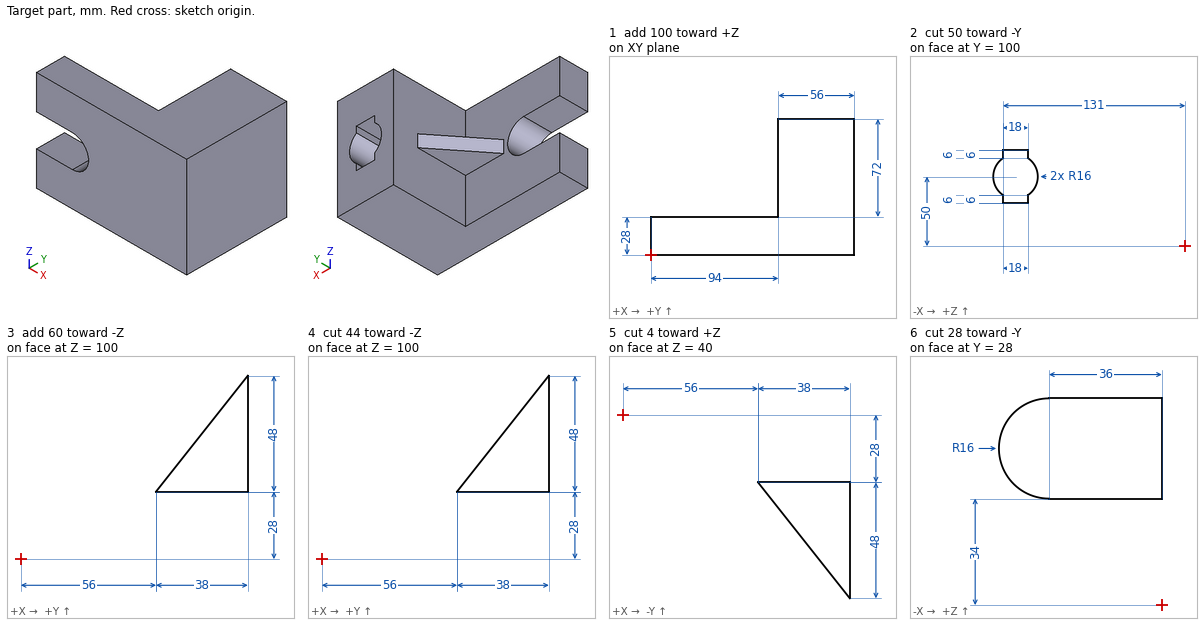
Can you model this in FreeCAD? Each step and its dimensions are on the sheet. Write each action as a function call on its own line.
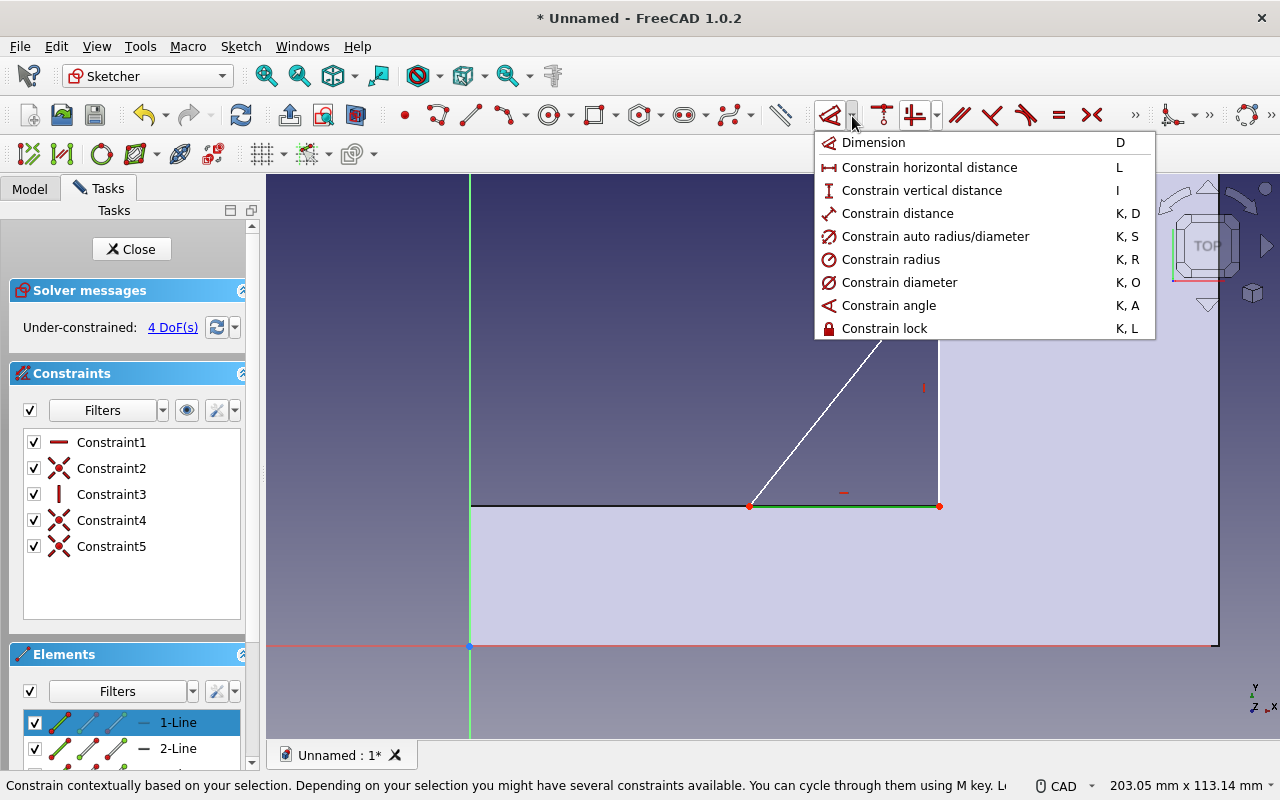
click(985, 168)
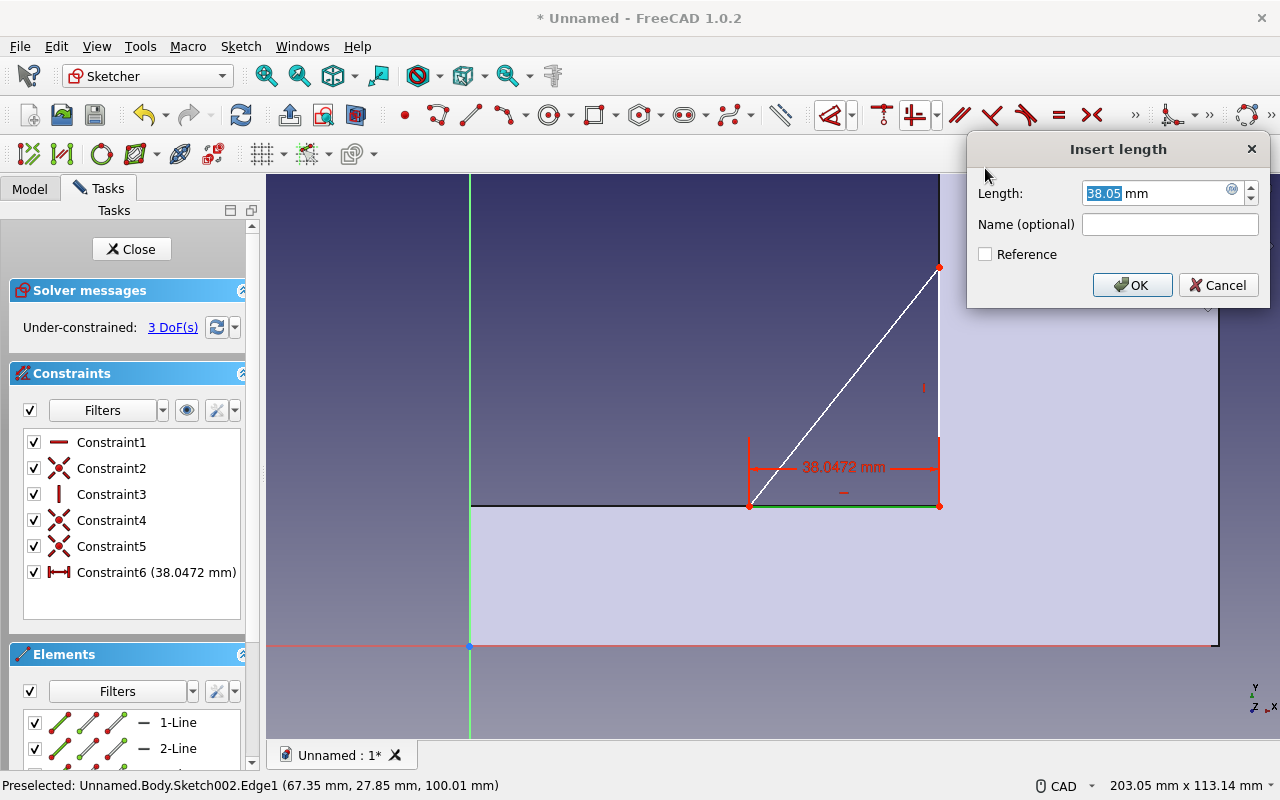
text(38)
key(Return)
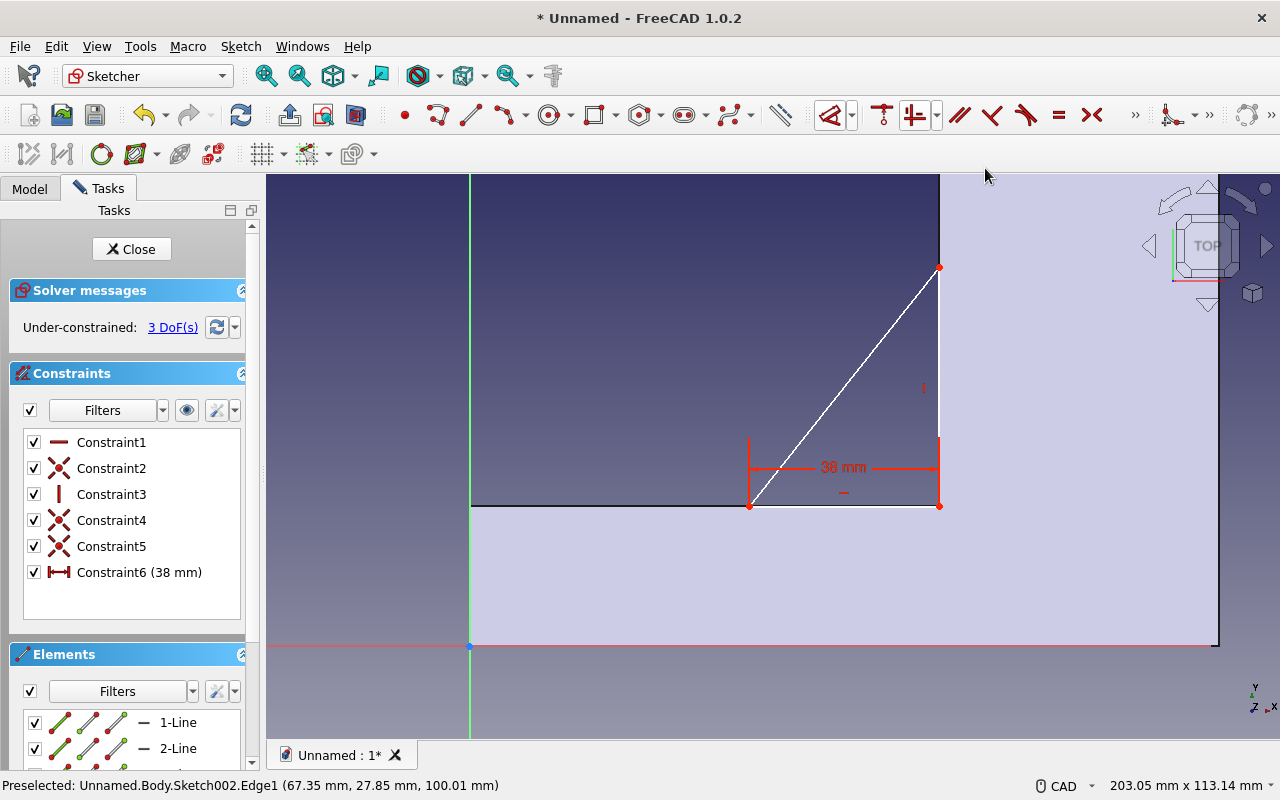
click(939, 435)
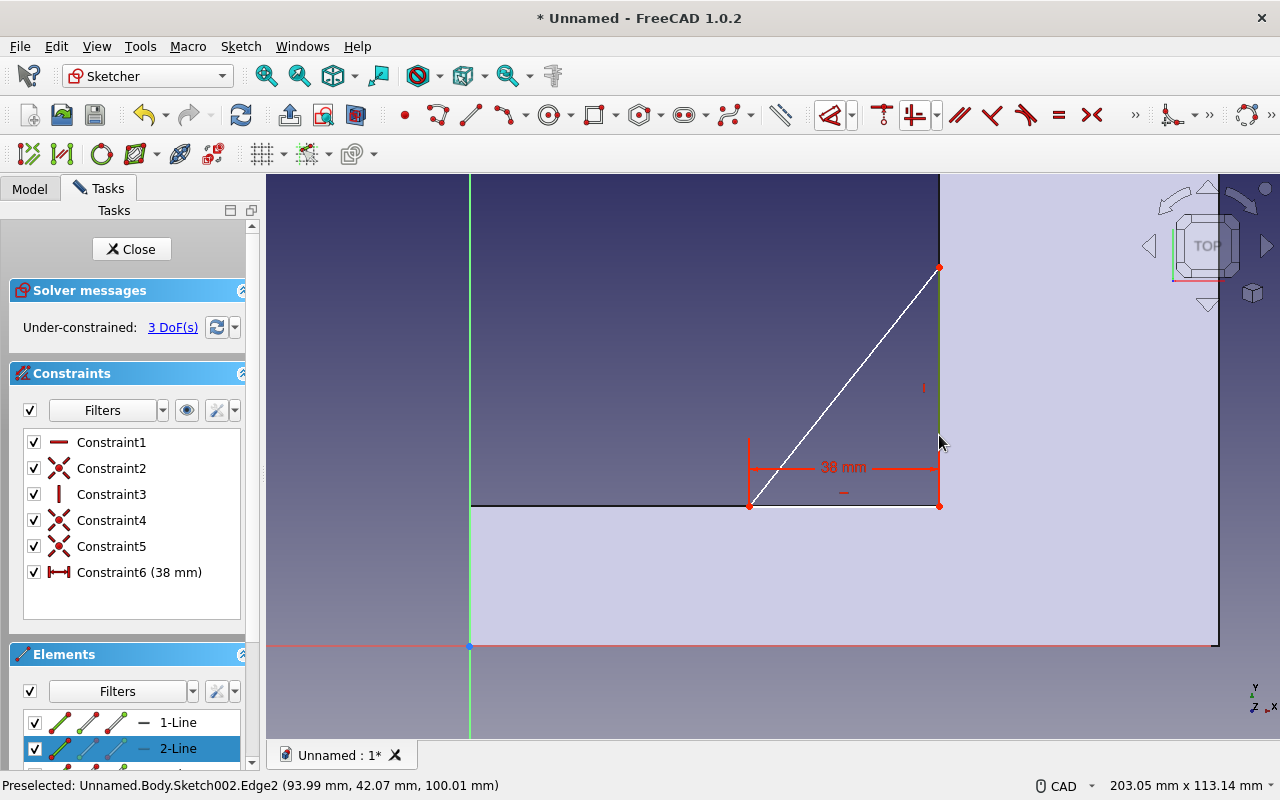
click(852, 116)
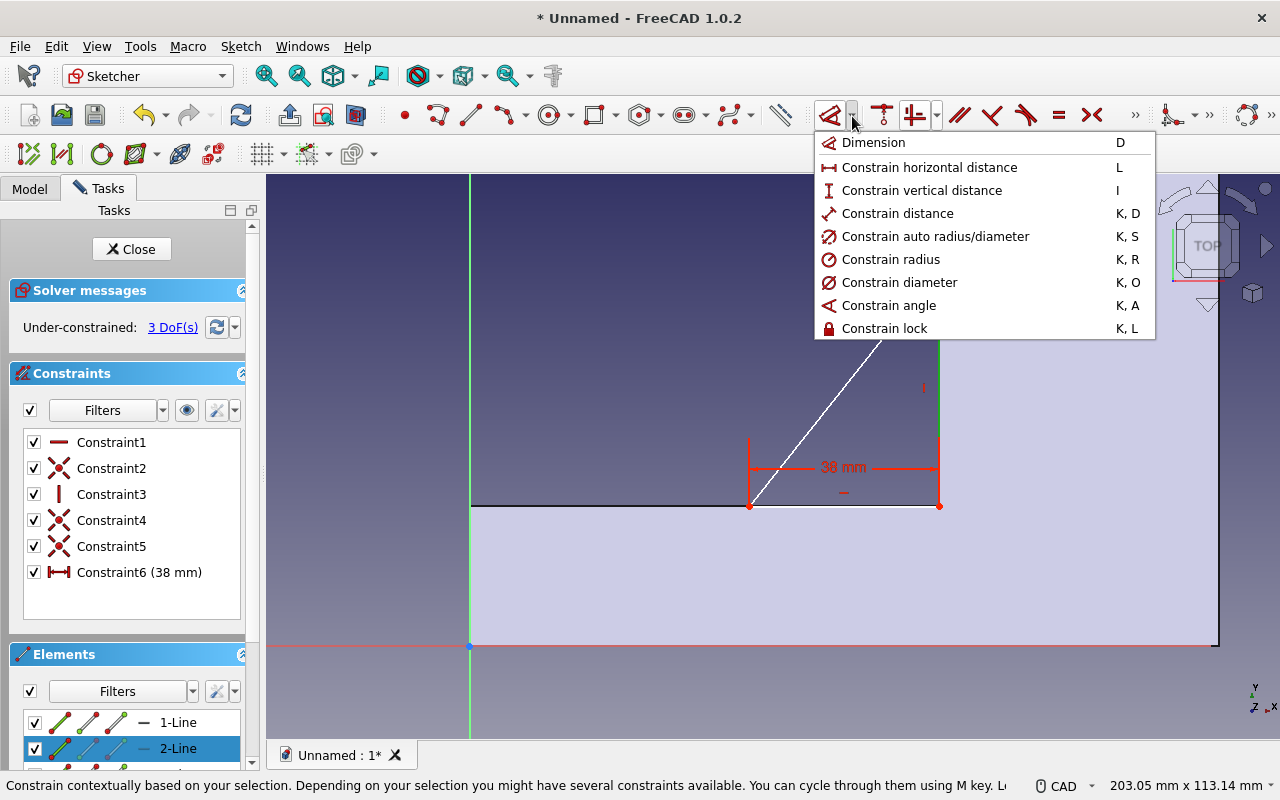
click(985, 190)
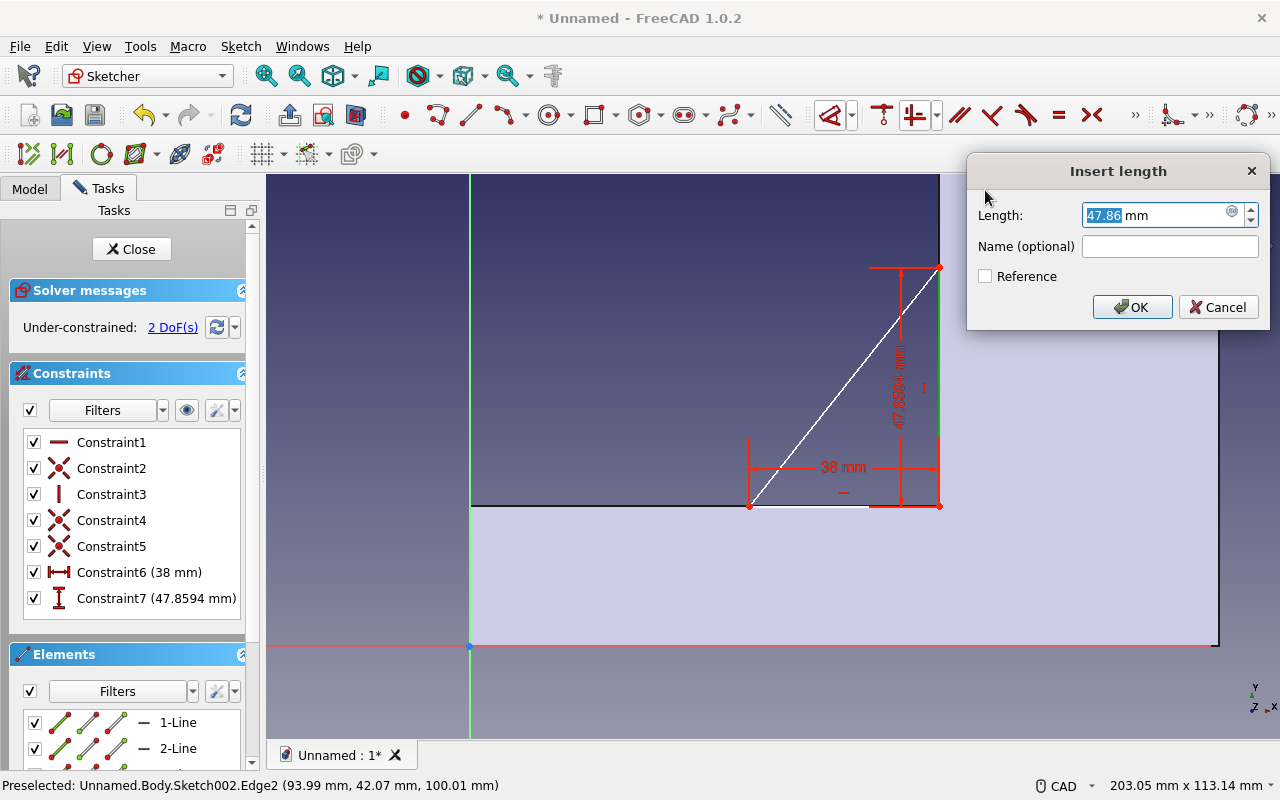
text(48)
key(Return)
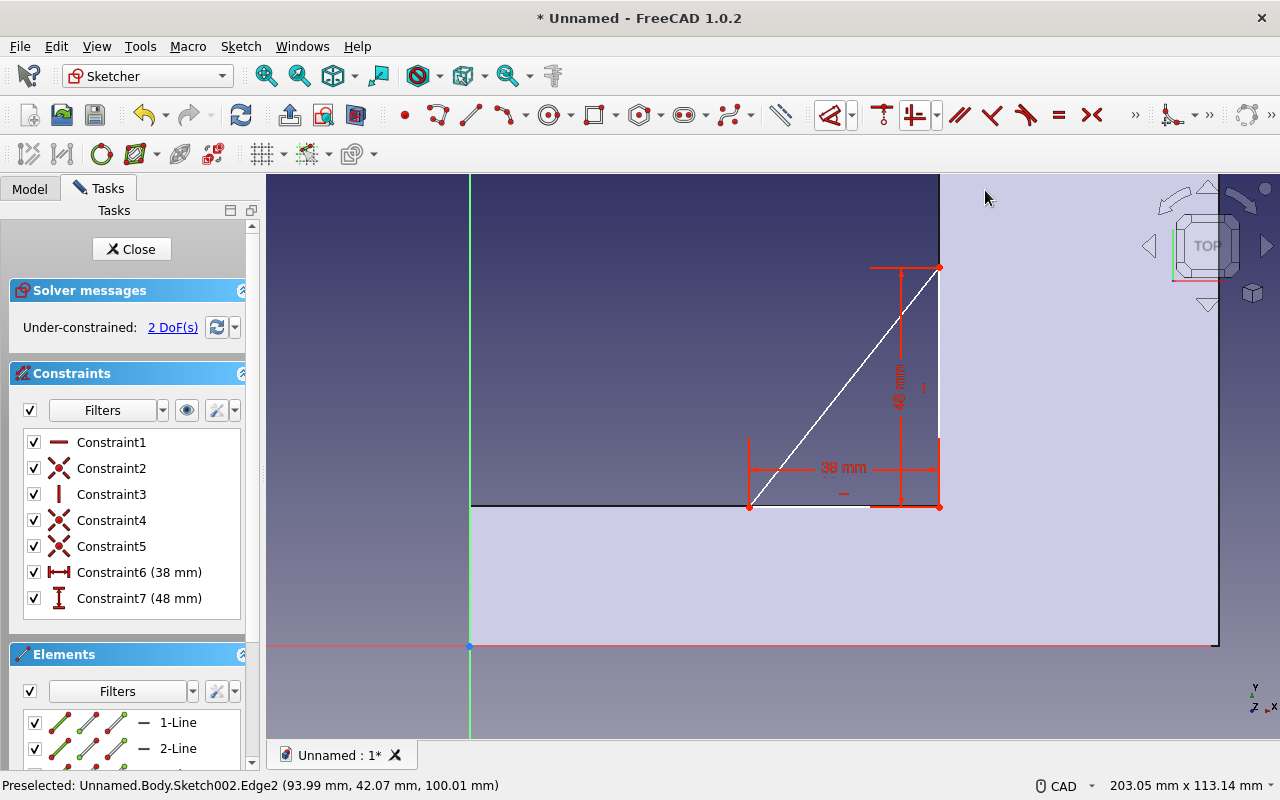
click(749, 507)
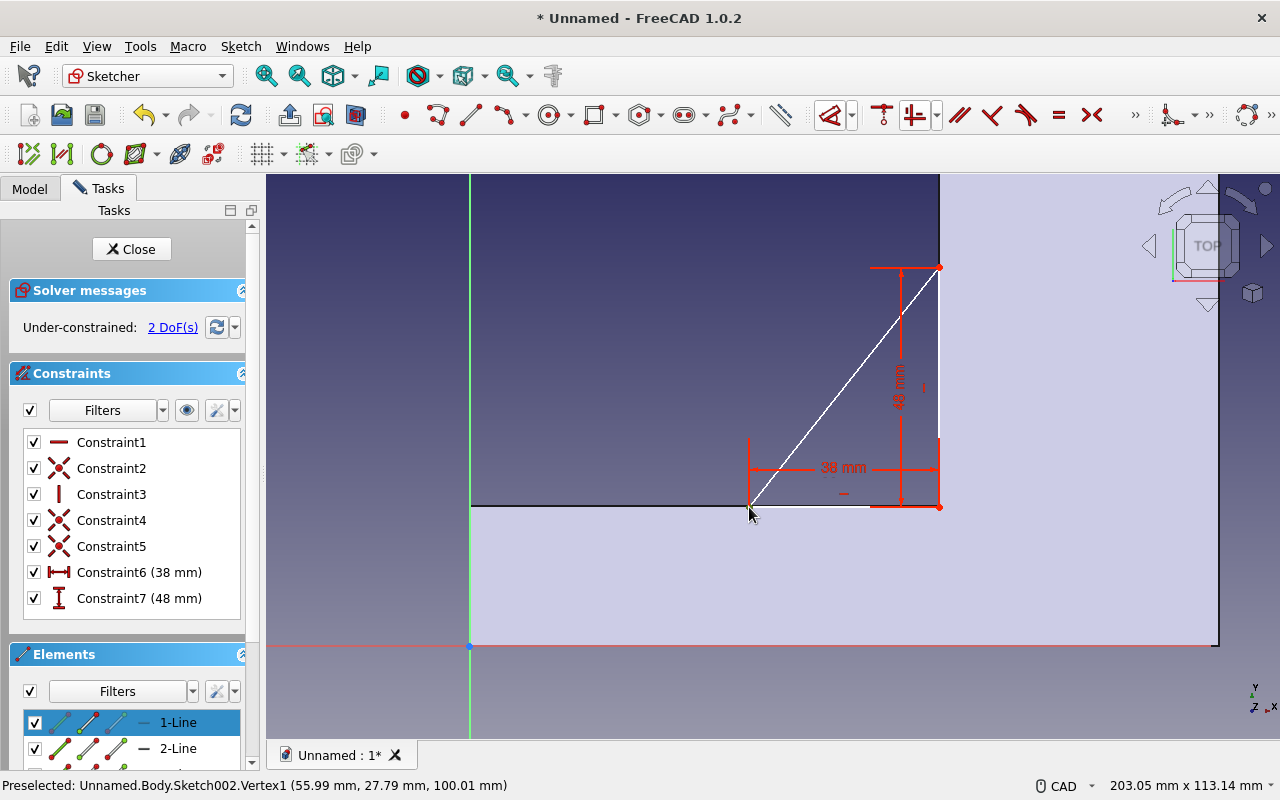
key(l)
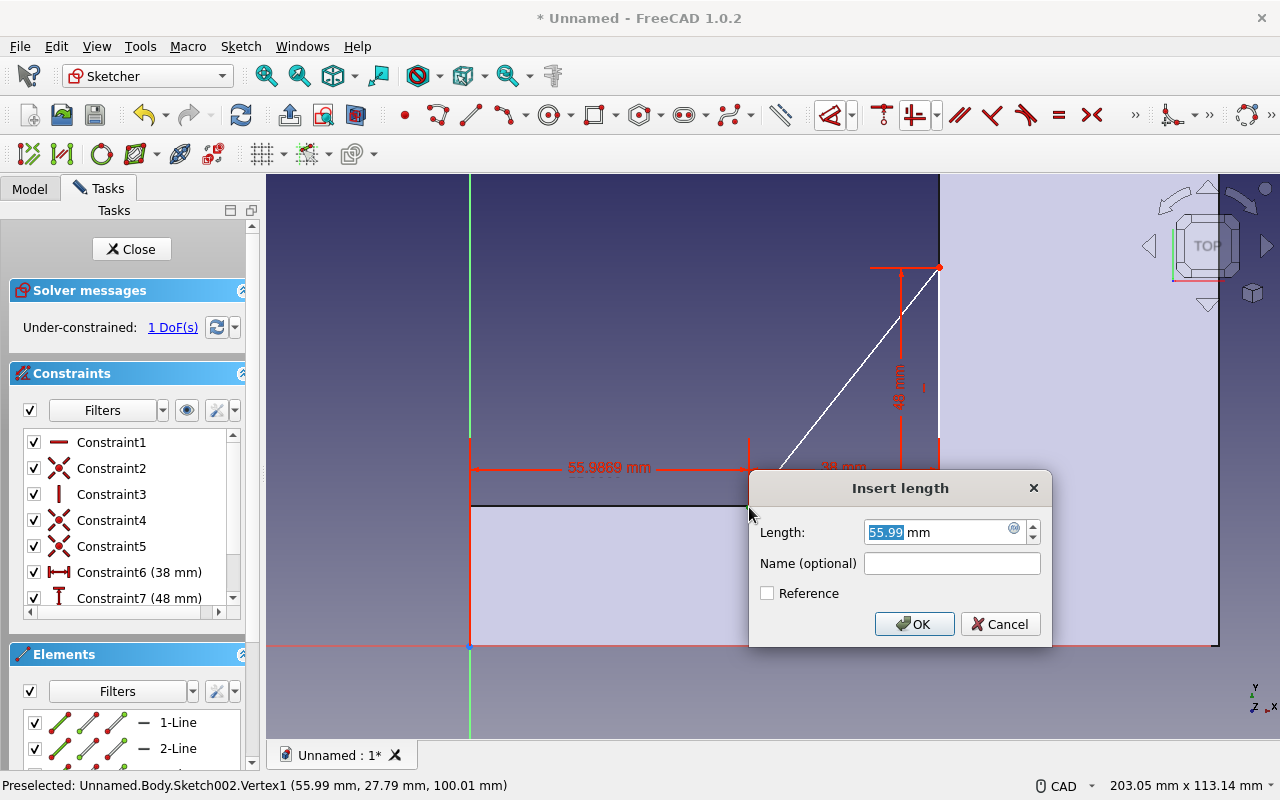
text(56)
key(Return)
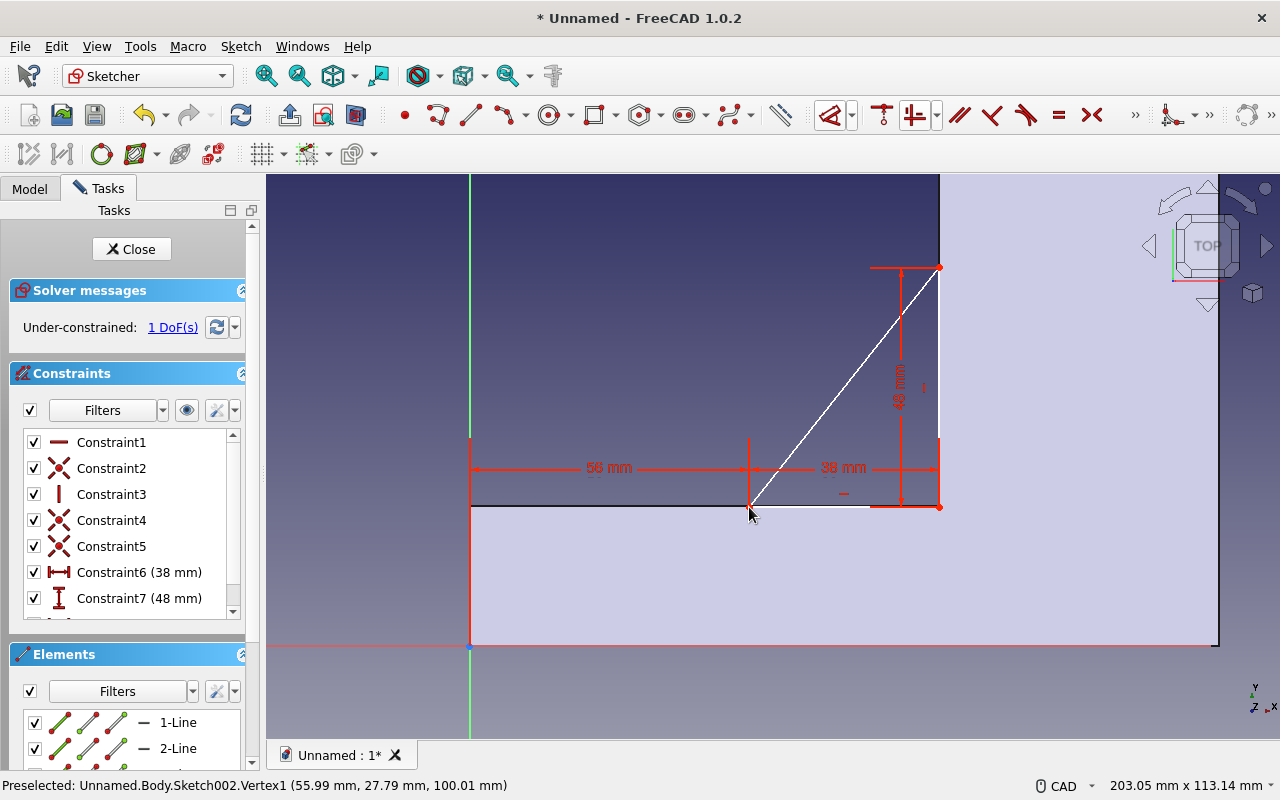
click(749, 507)